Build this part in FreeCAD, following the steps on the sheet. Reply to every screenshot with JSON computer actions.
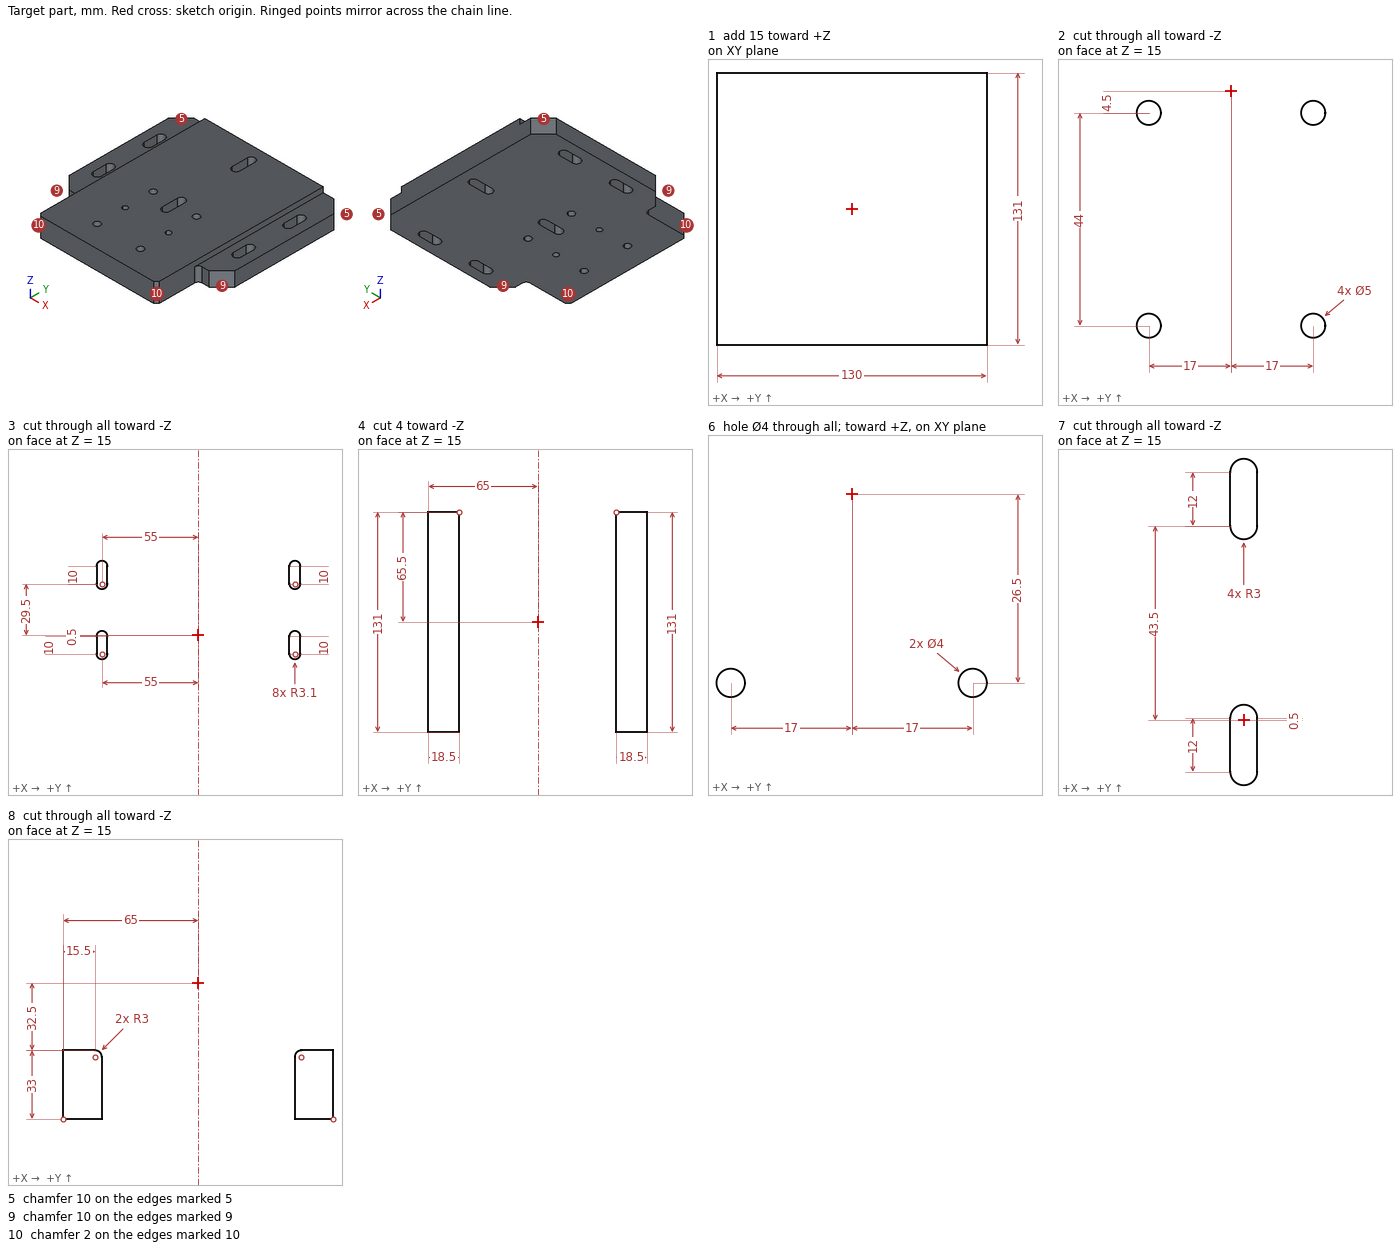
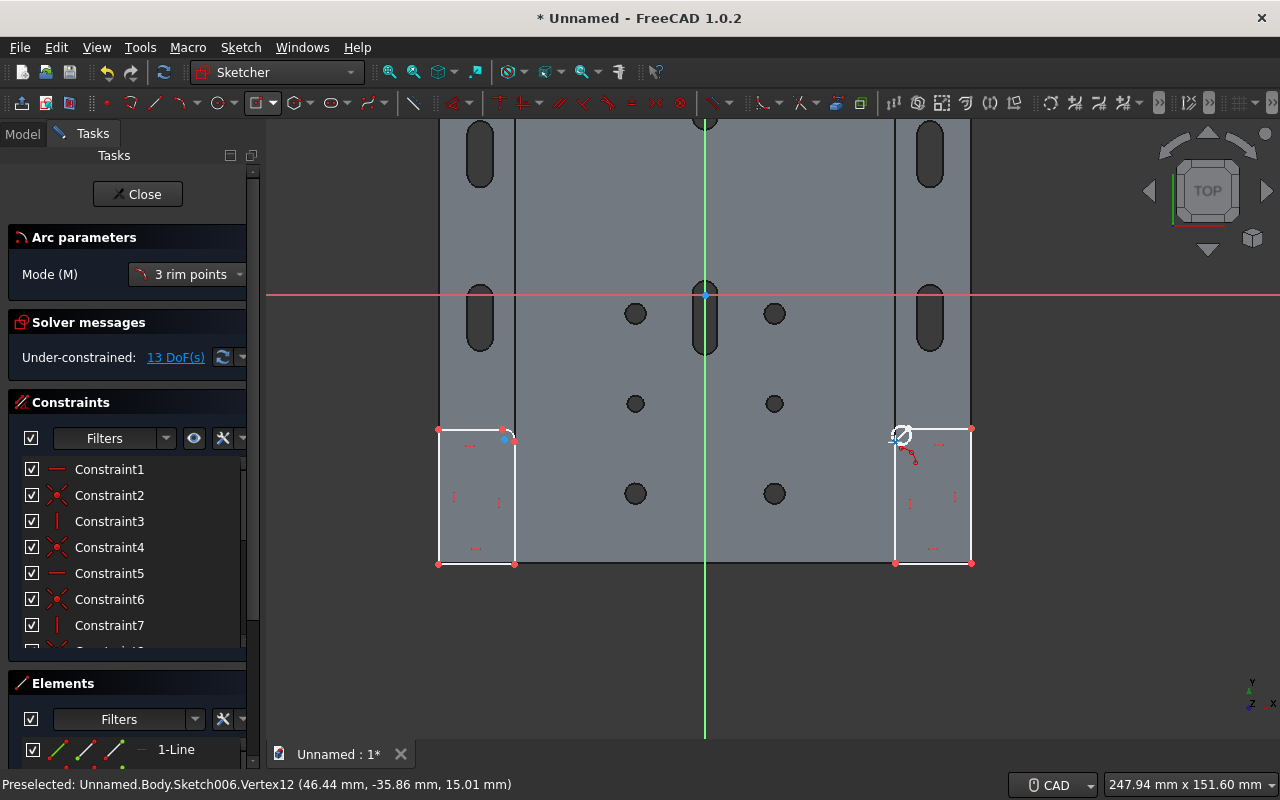
{"action": "scroll", "coordinate": [899, 432], "scroll_direction": "up", "scroll_amount": 8}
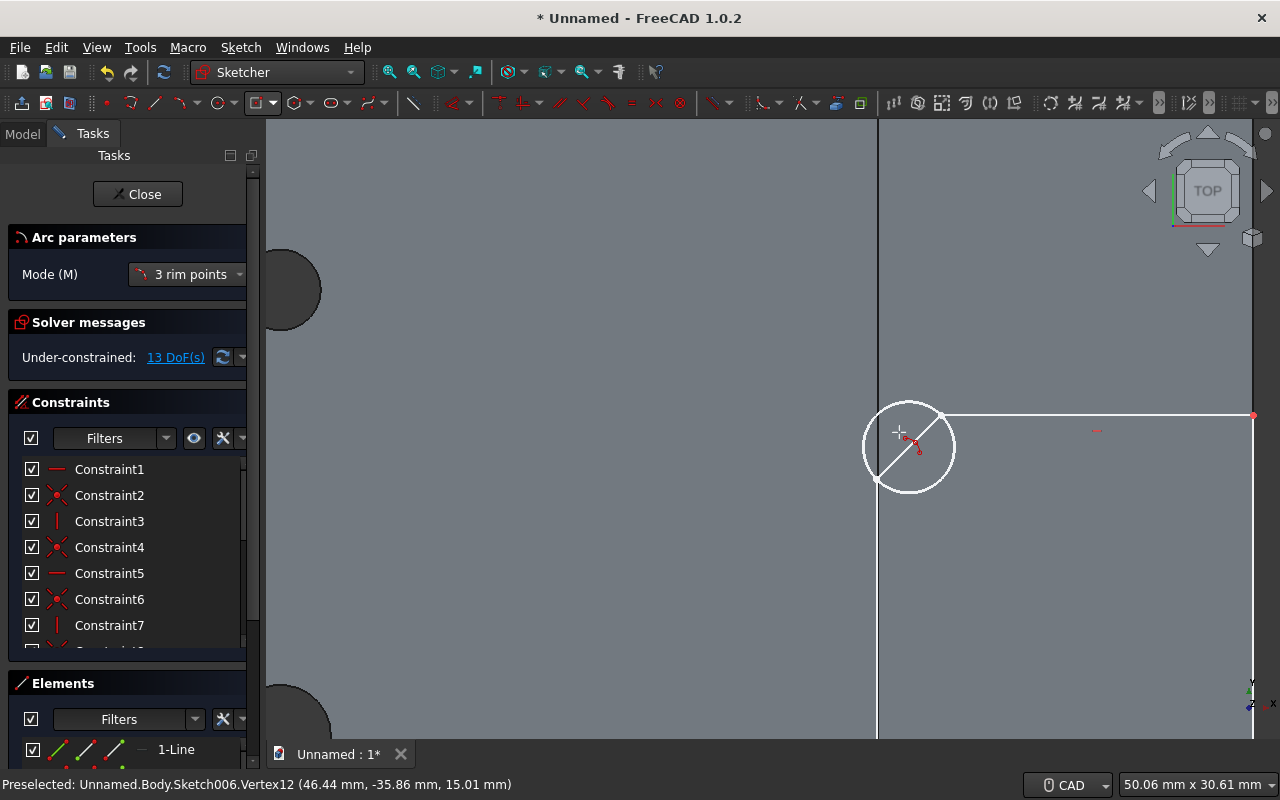
{"action": "left_click", "coordinate": [896, 429]}
{"action": "key", "text": "Escape"}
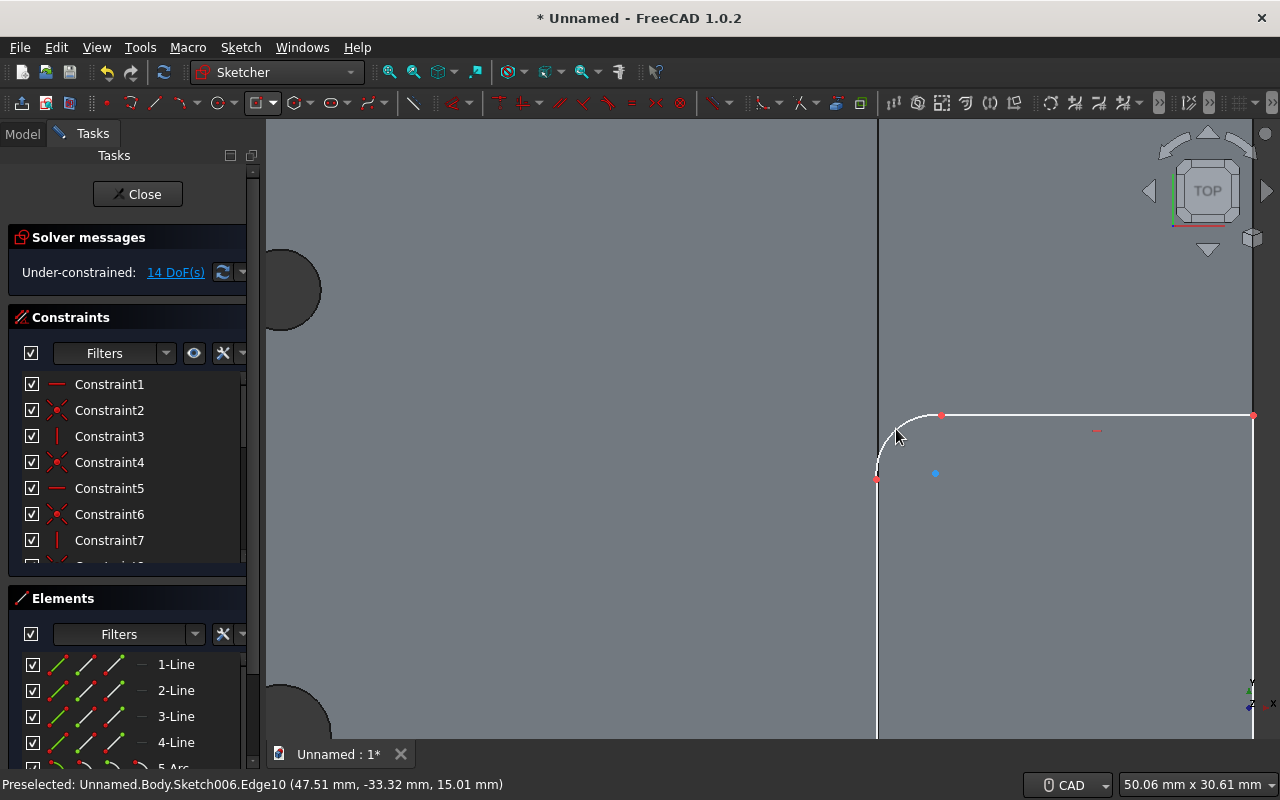
{"action": "scroll", "coordinate": [899, 432], "scroll_direction": "down", "scroll_amount": 8}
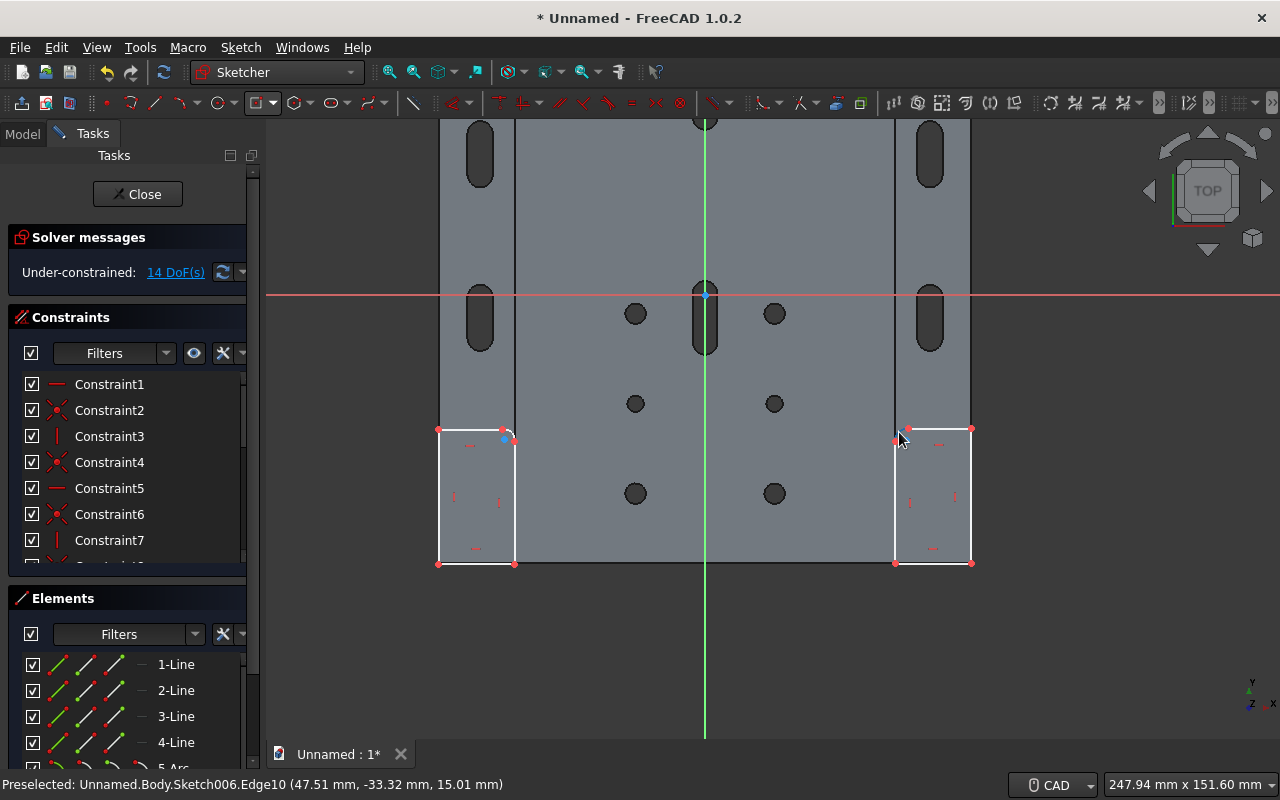
{"action": "left_click", "coordinate": [483, 430]}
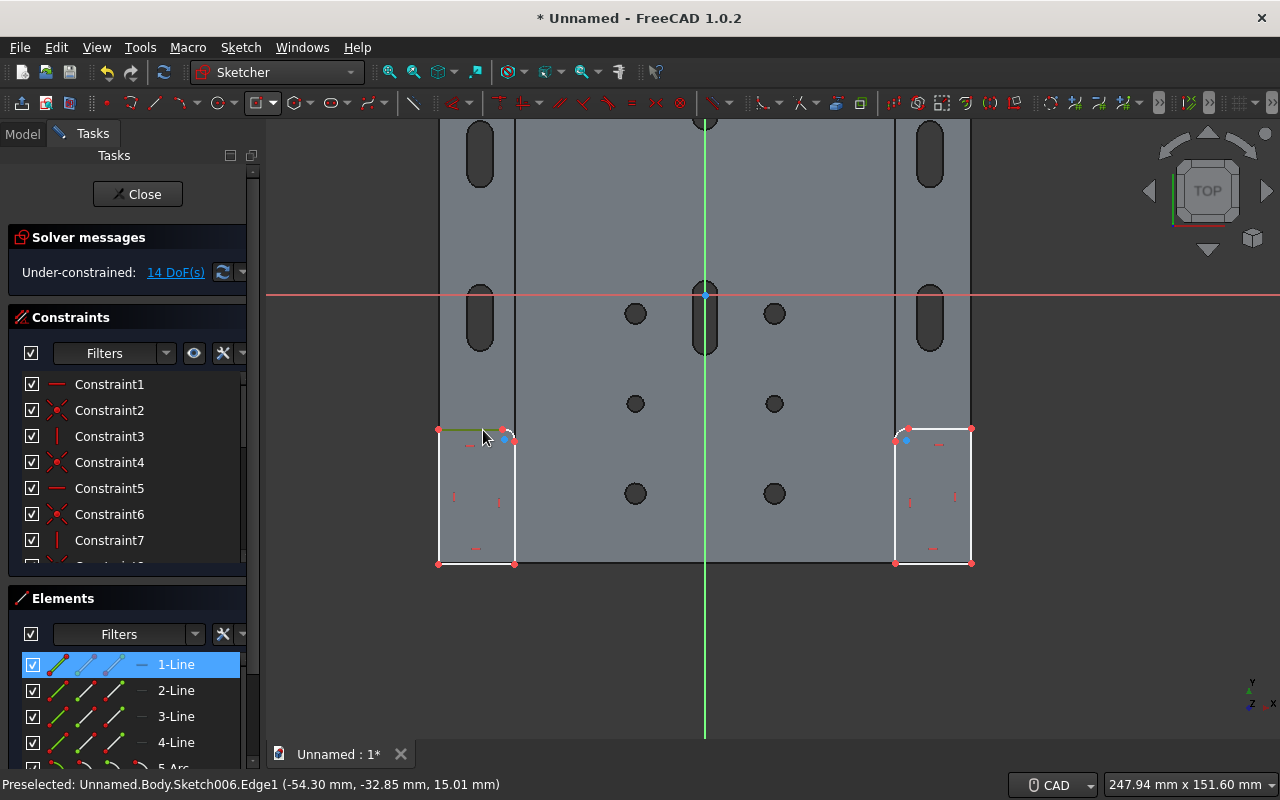
{"action": "scroll", "coordinate": [512, 432], "scroll_direction": "up", "scroll_amount": 2}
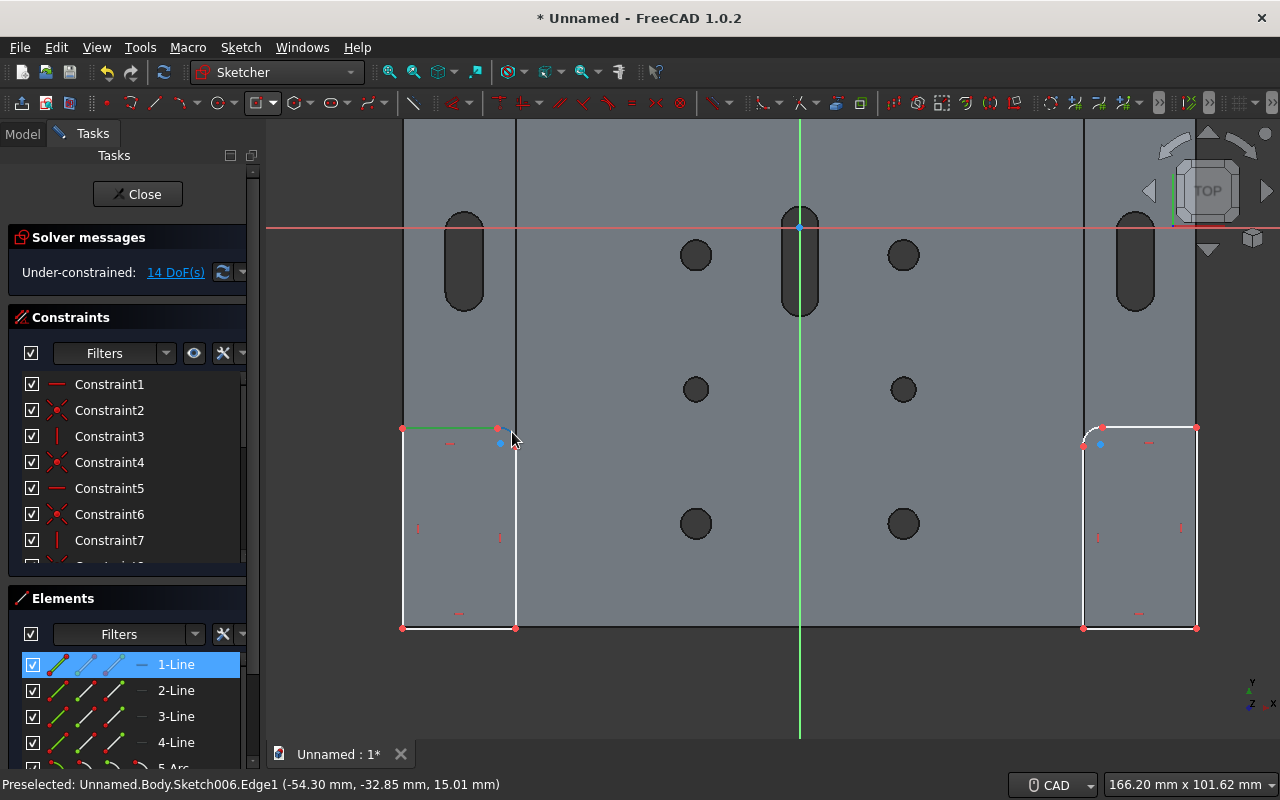
{"action": "left_click", "coordinate": [511, 432]}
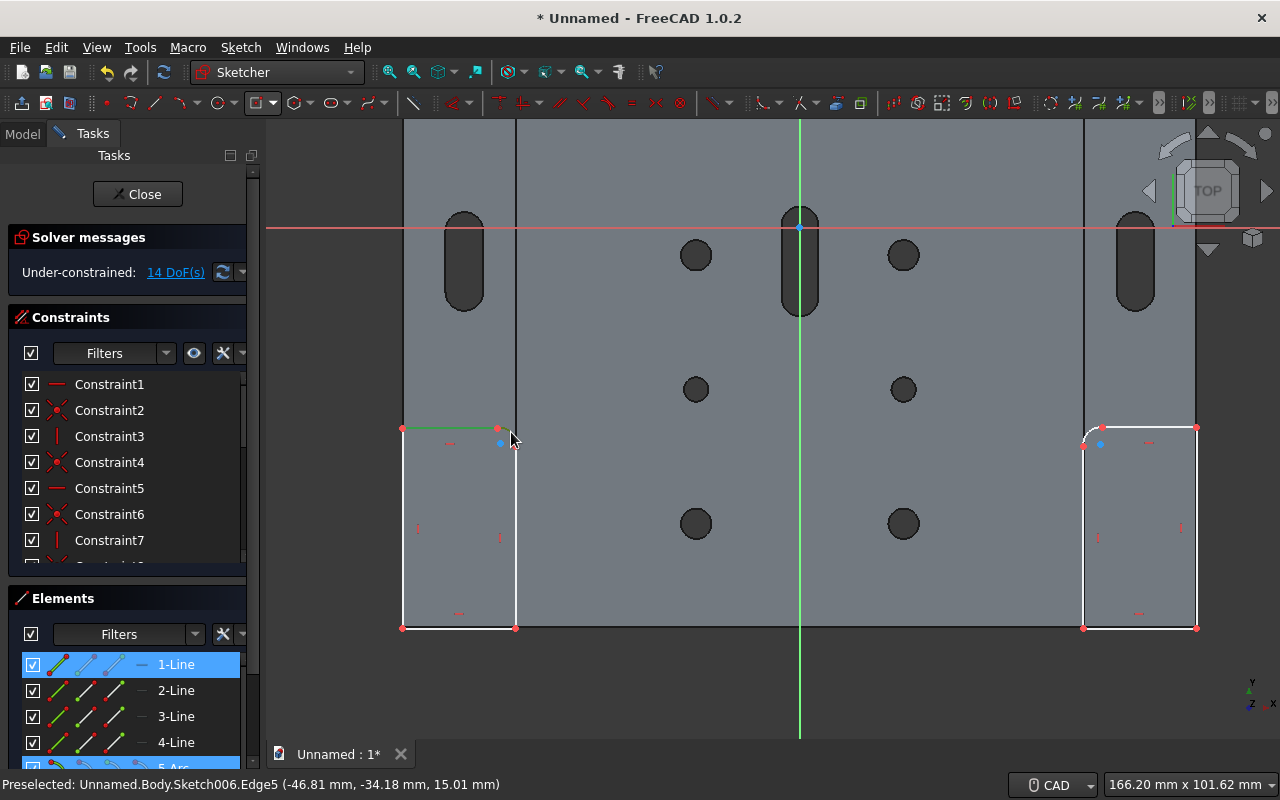
{"action": "left_click", "coordinate": [608, 104]}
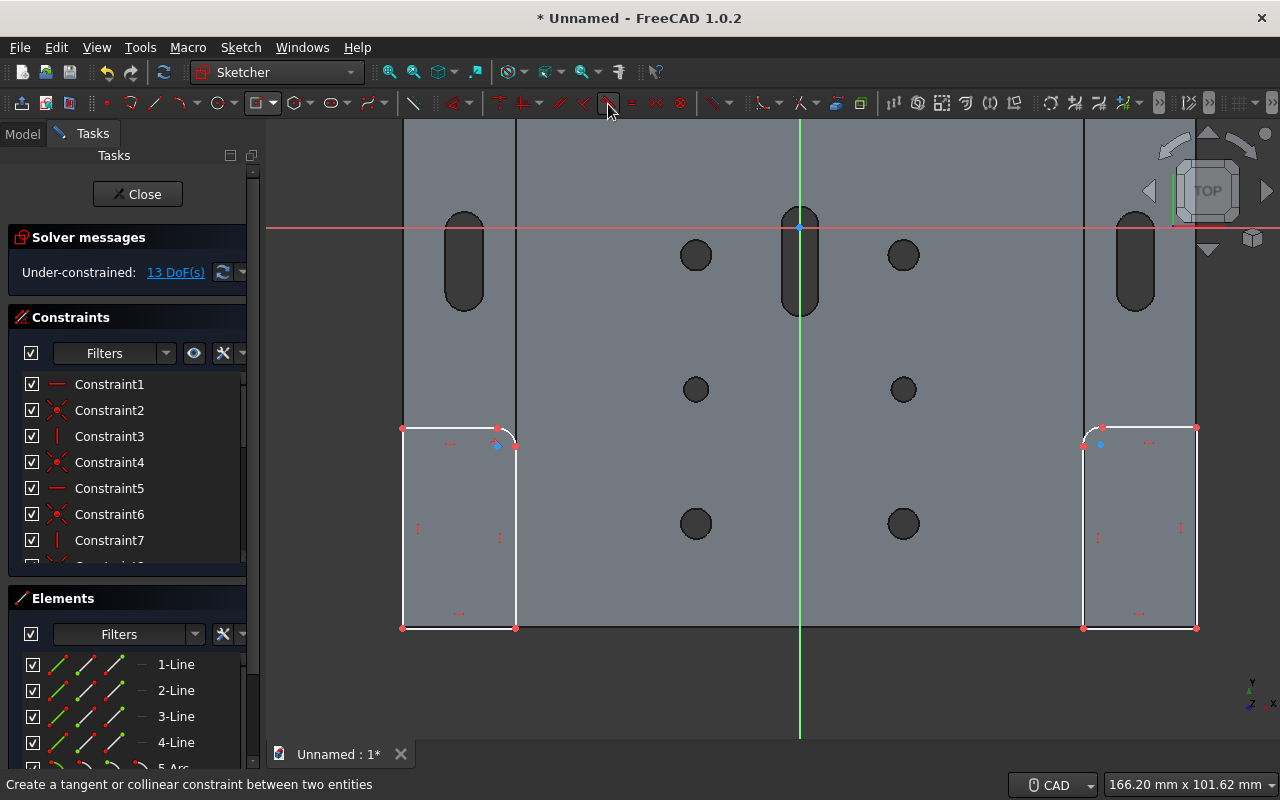
{"action": "left_click", "coordinate": [516, 574]}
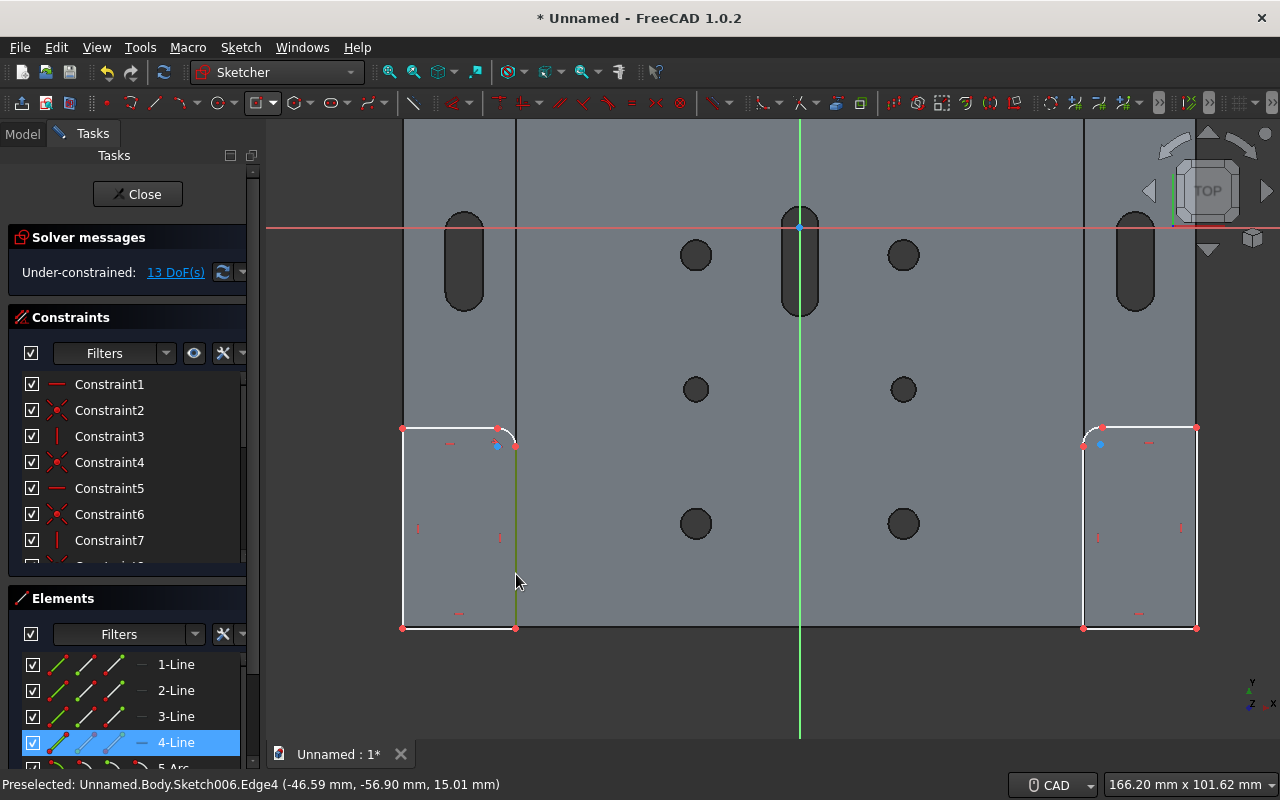
{"action": "left_click", "coordinate": [510, 434]}